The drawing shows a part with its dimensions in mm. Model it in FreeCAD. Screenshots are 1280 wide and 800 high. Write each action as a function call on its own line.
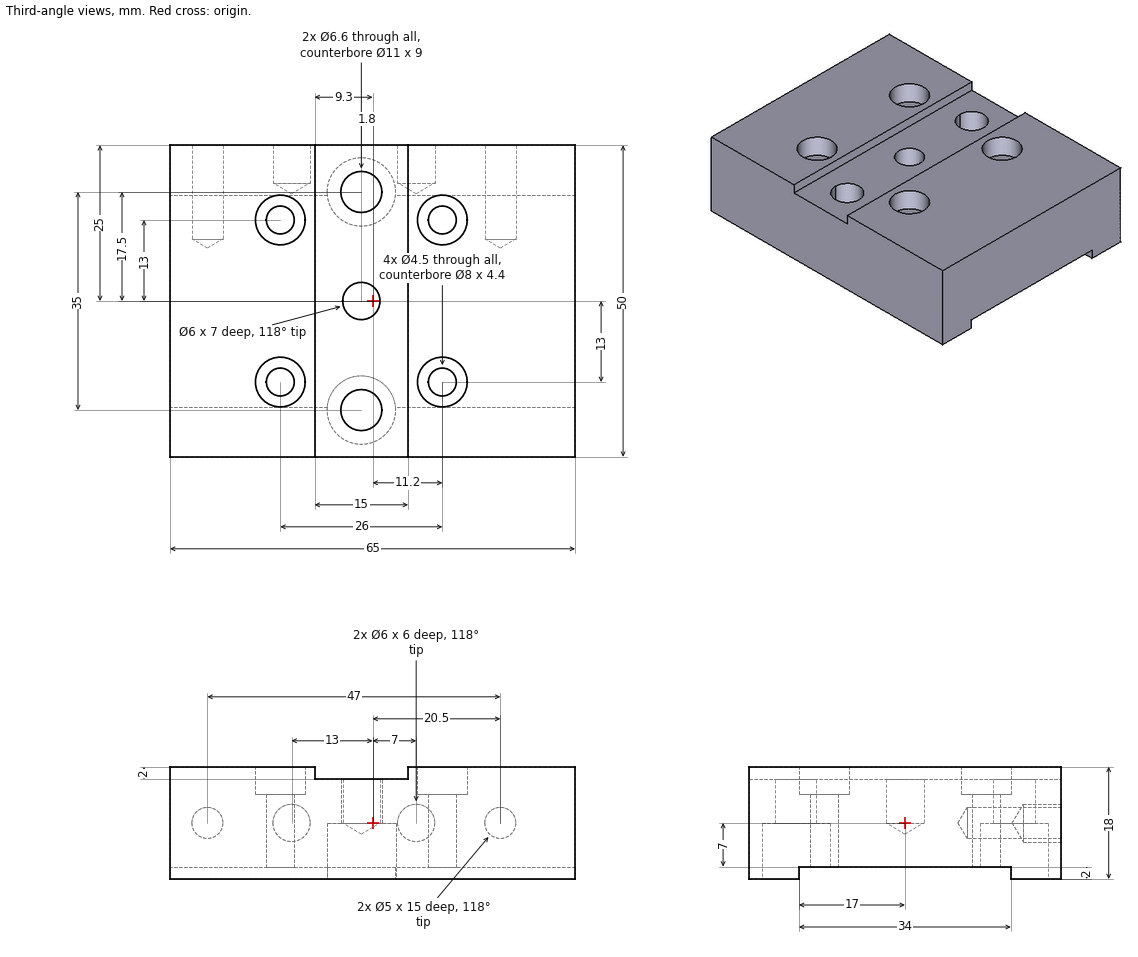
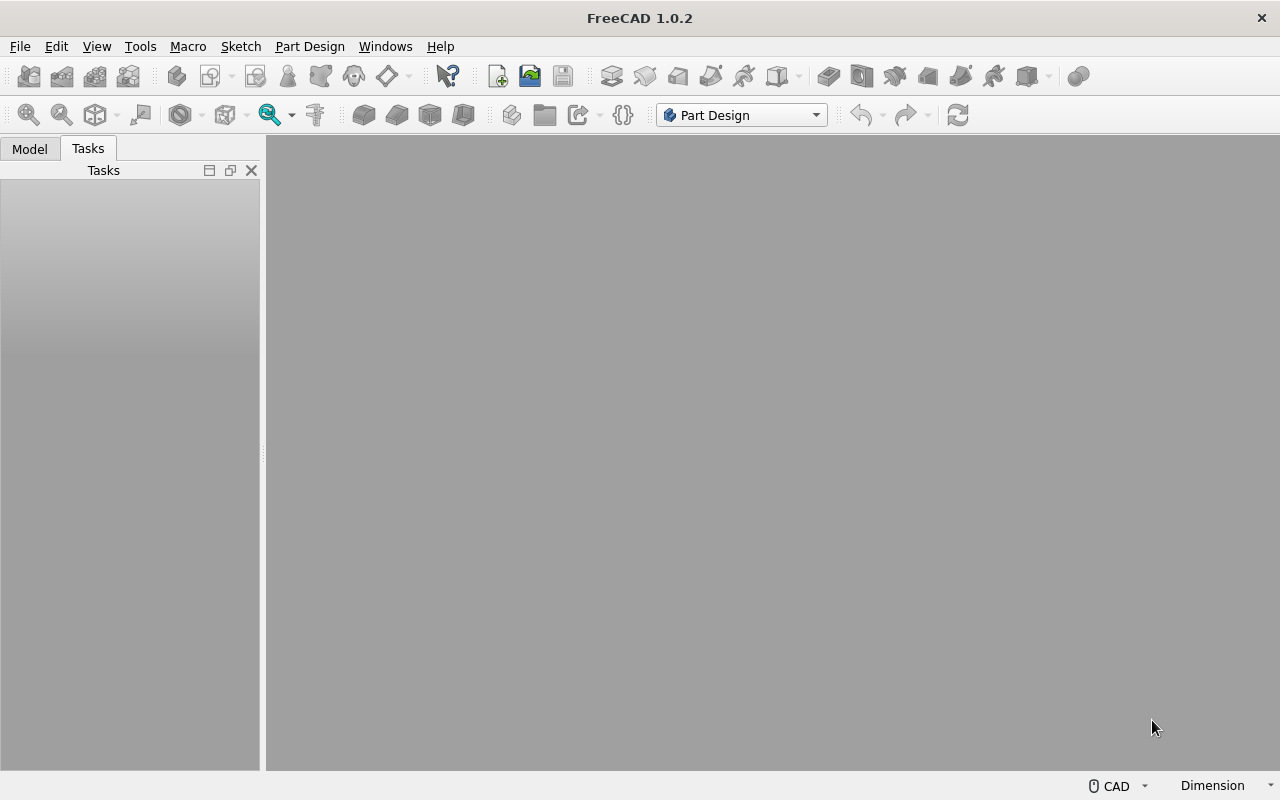
key(ctrl+n)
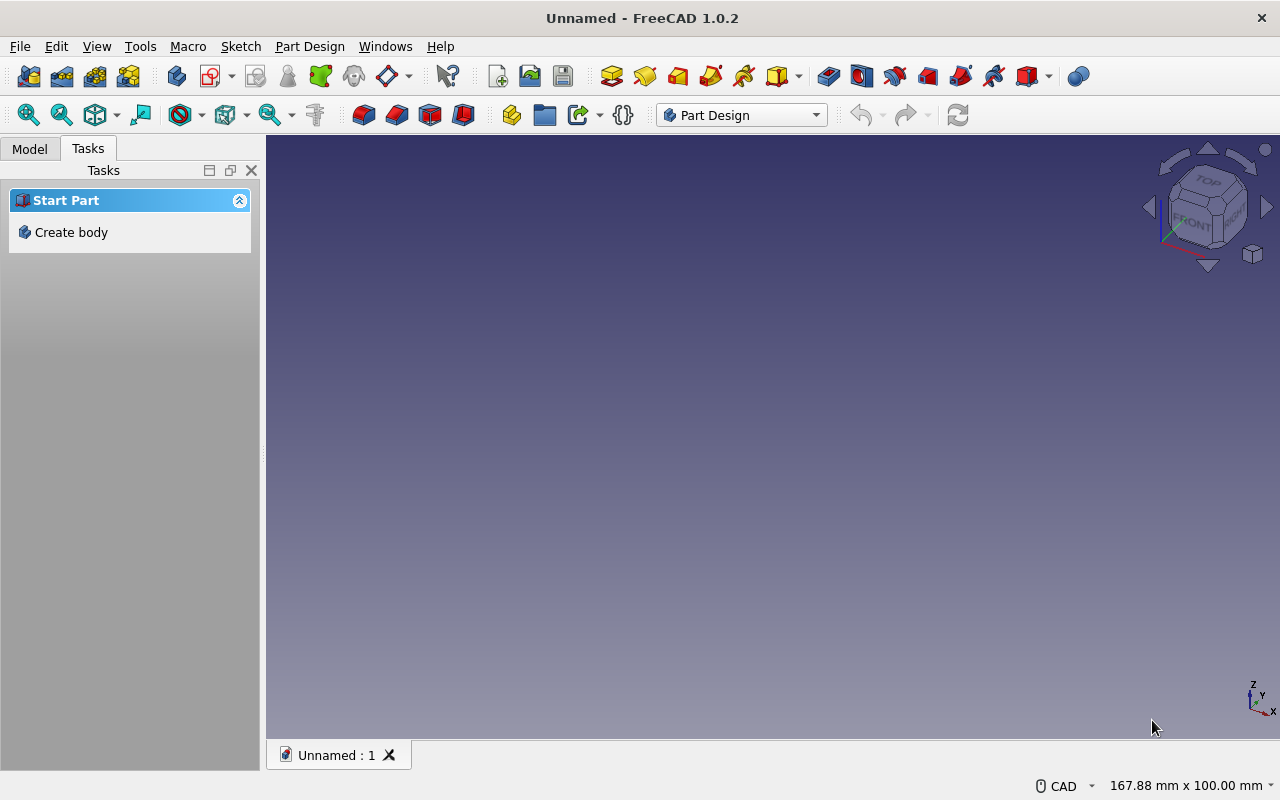
click(210, 76)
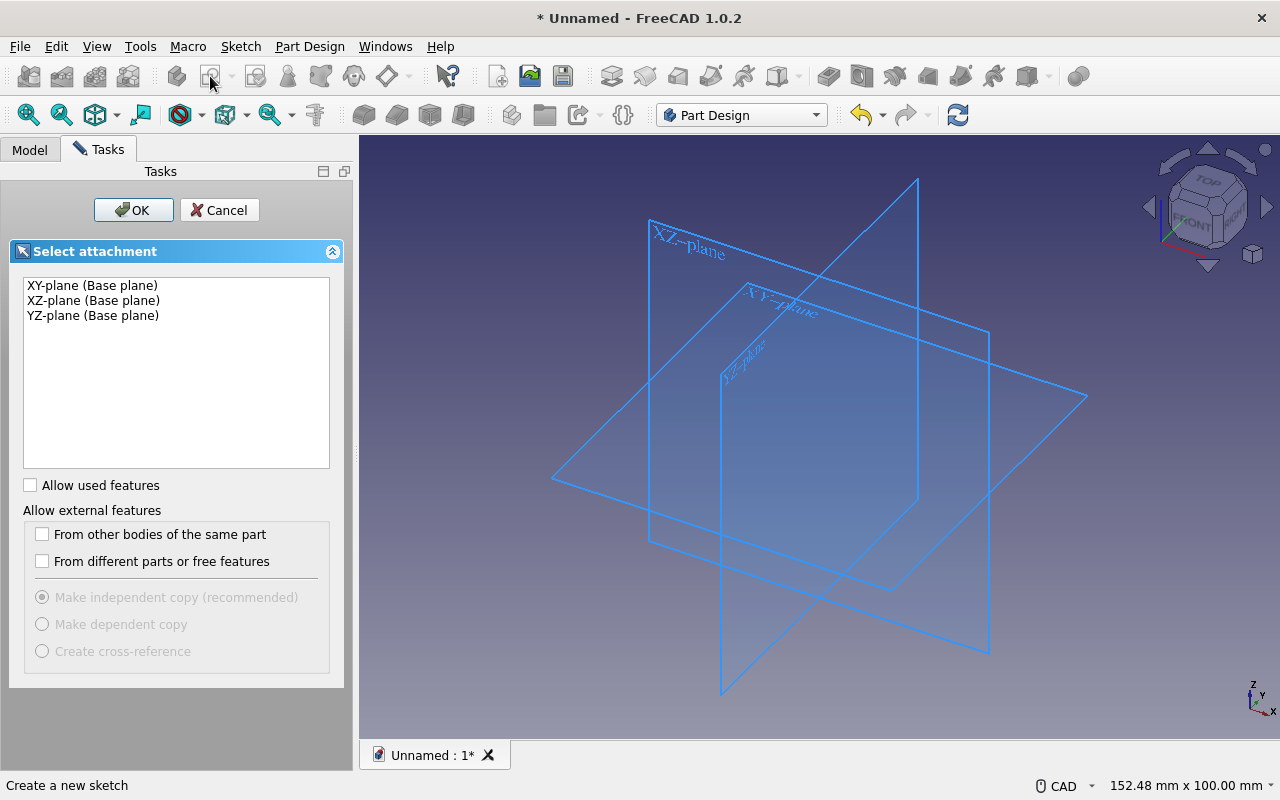
click(84, 286)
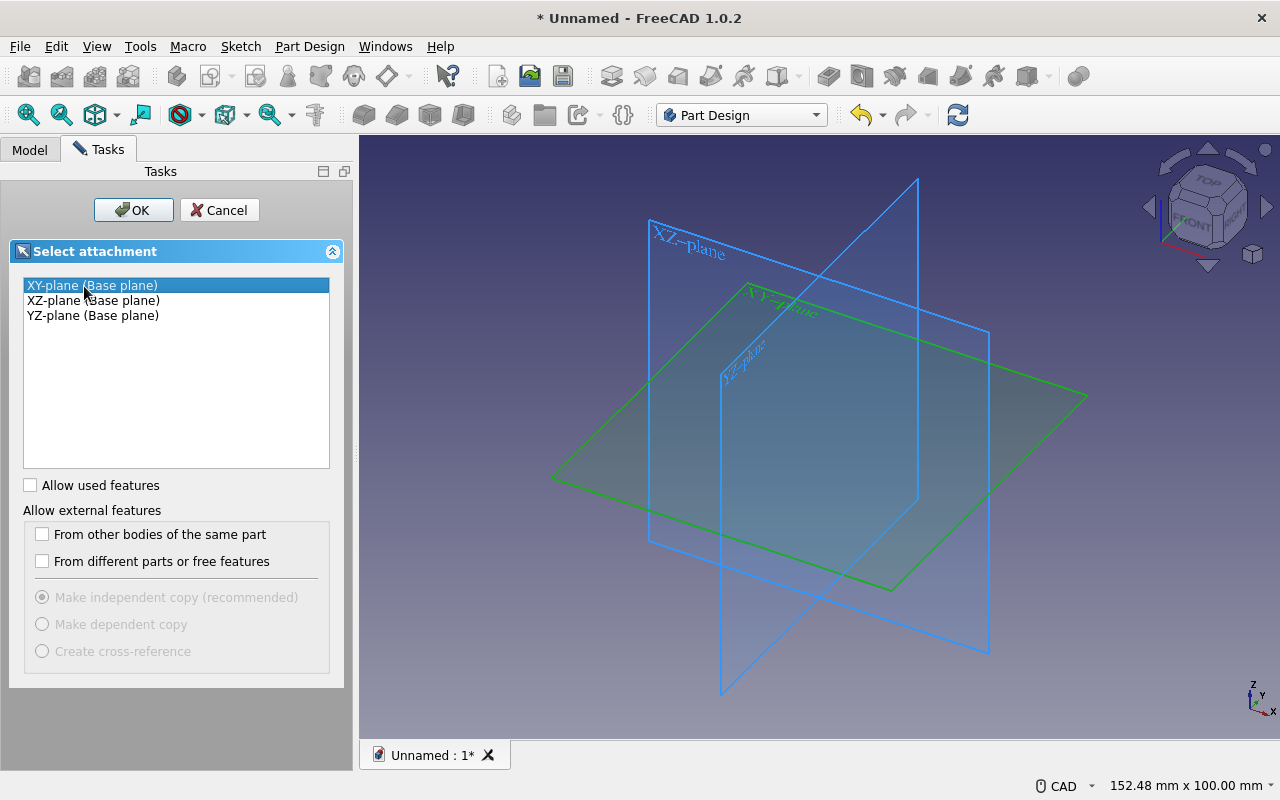
click(134, 210)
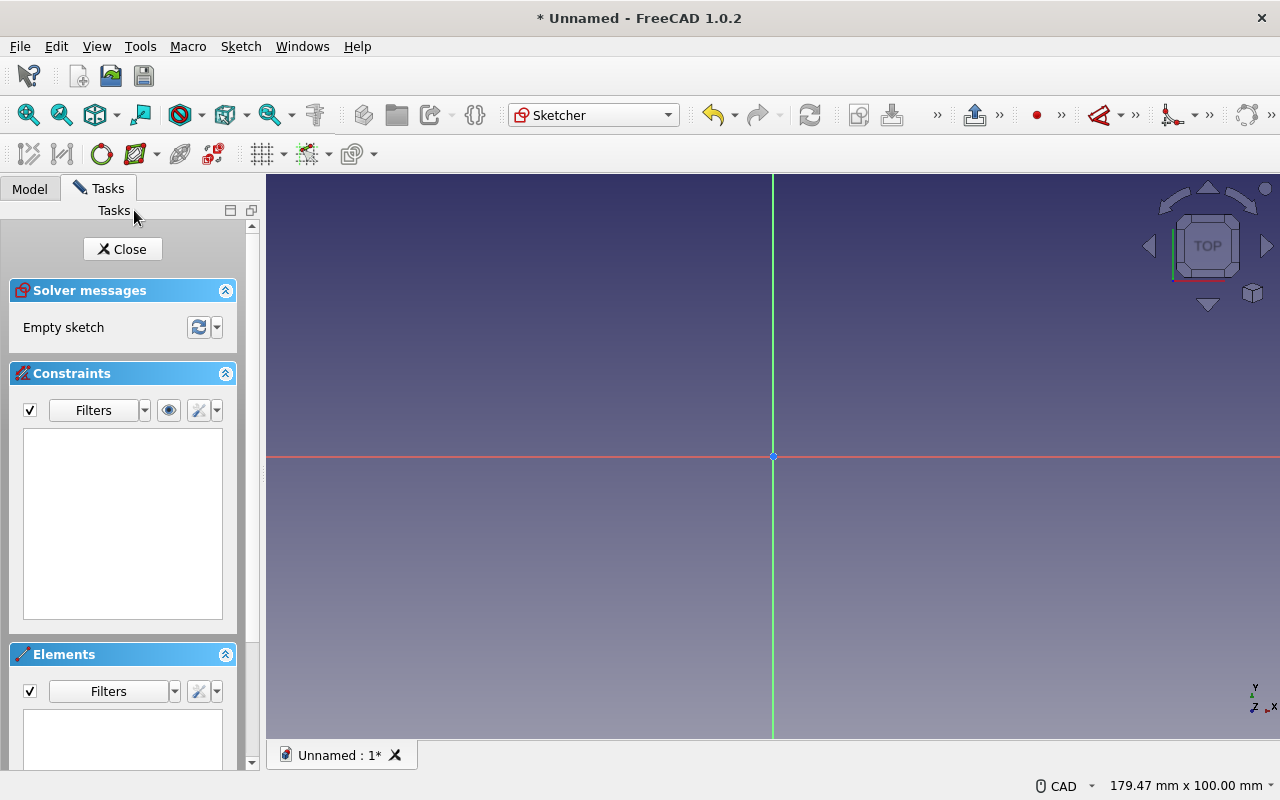
key(g)
key(v)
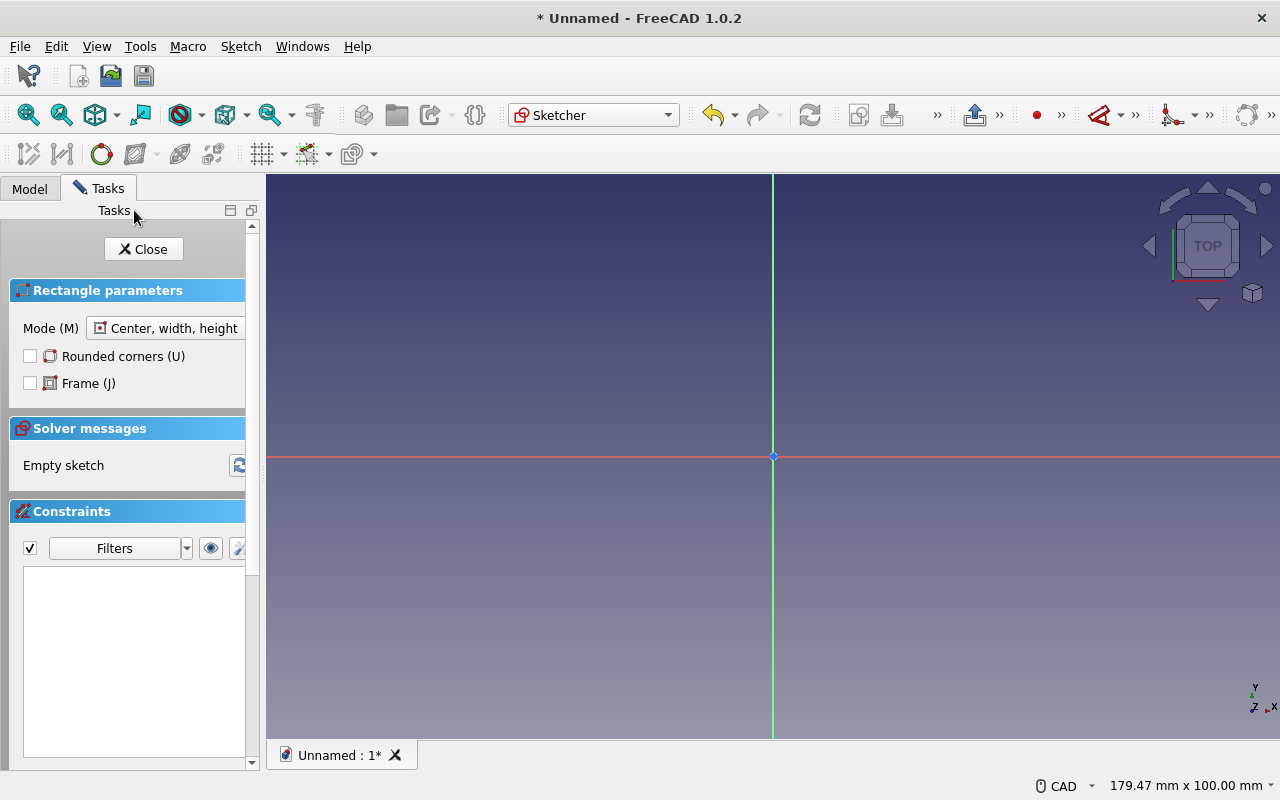
click(773, 456)
move(957, 315)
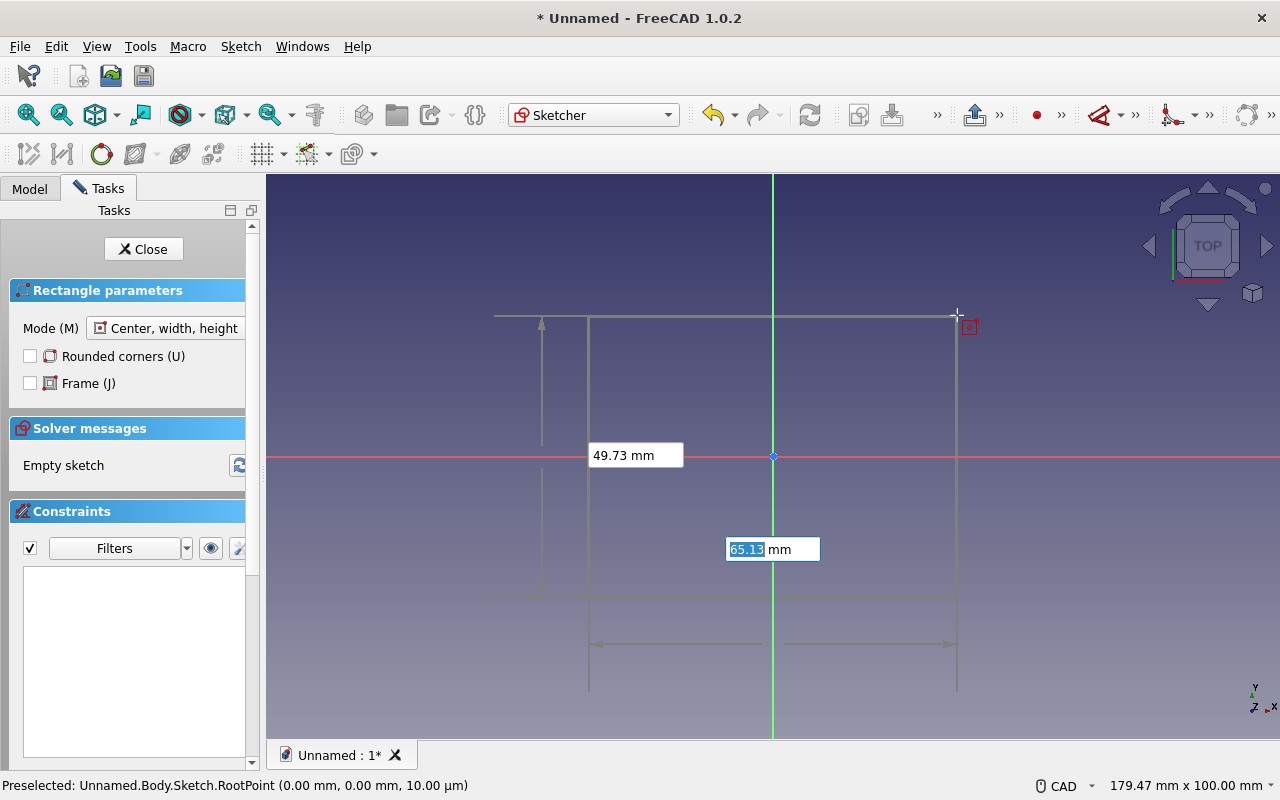
text(65)
key(Tab)
text(50)
key(Return)
key(Escape)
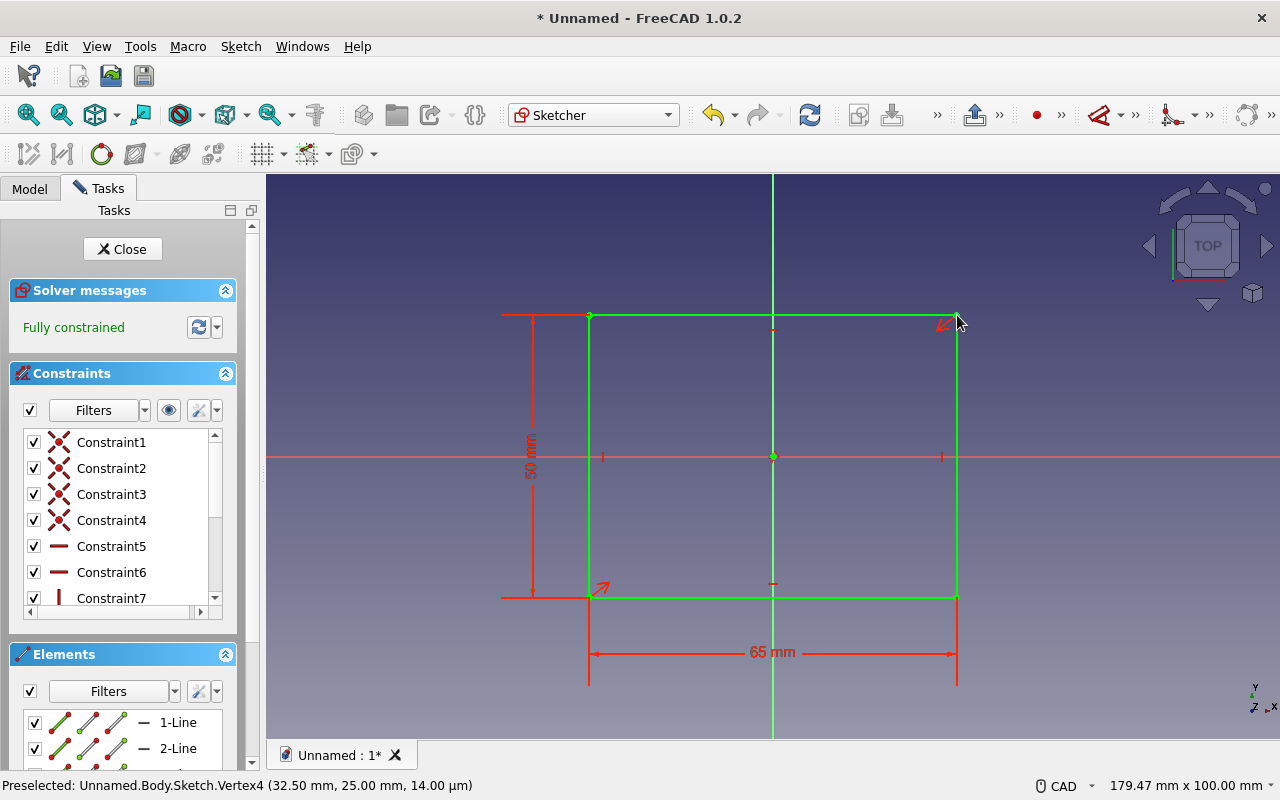
click(123, 249)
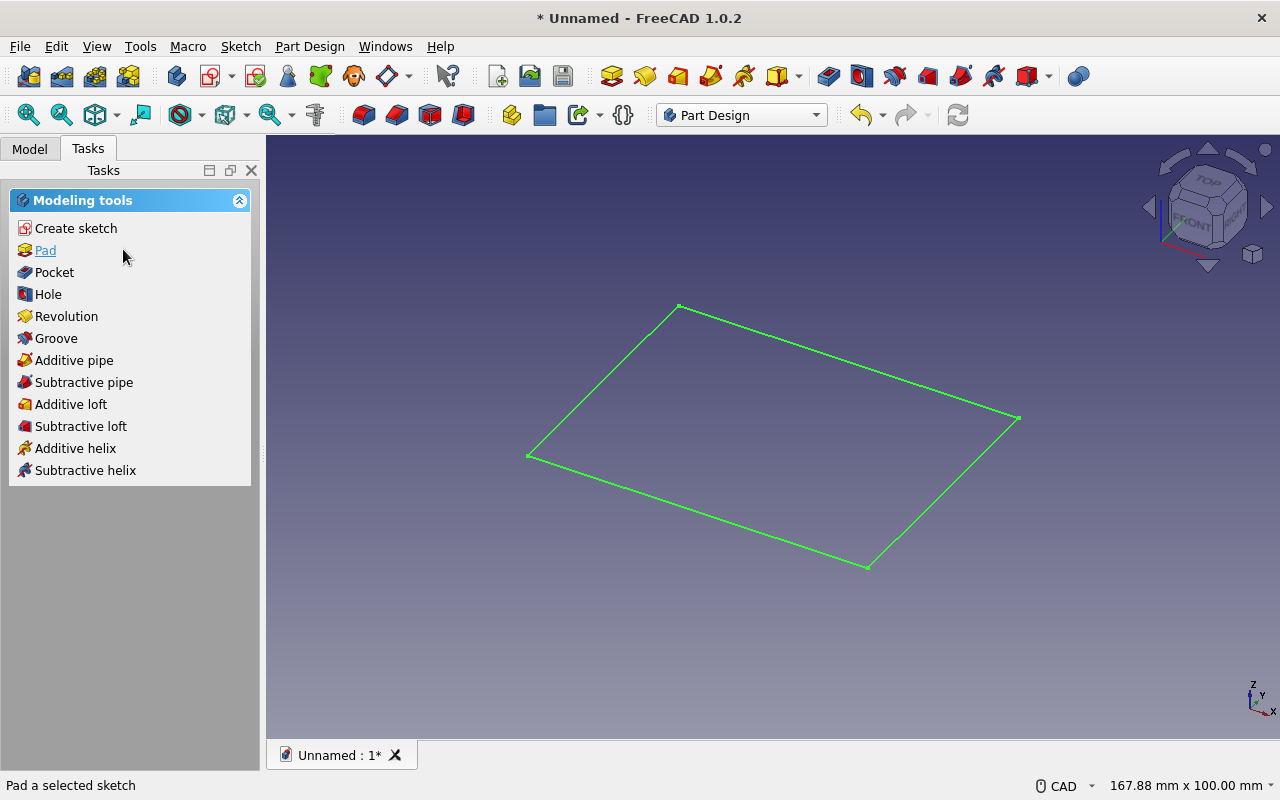
click(612, 76)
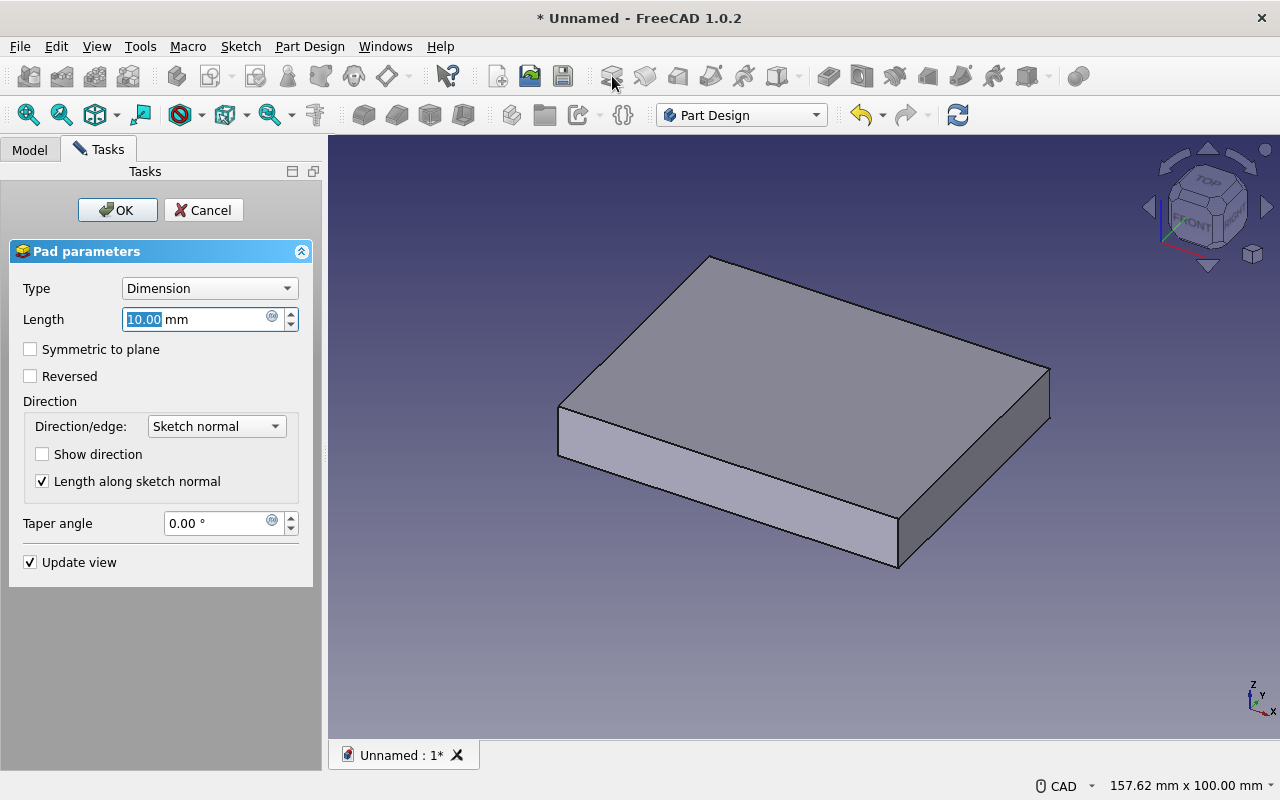
text(18)
key(Tab)